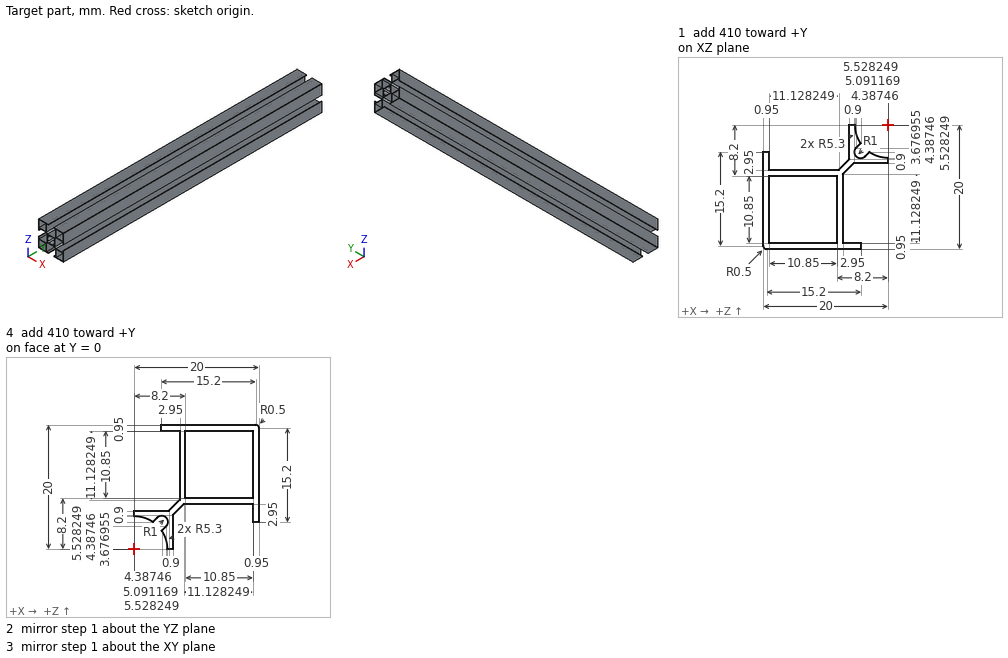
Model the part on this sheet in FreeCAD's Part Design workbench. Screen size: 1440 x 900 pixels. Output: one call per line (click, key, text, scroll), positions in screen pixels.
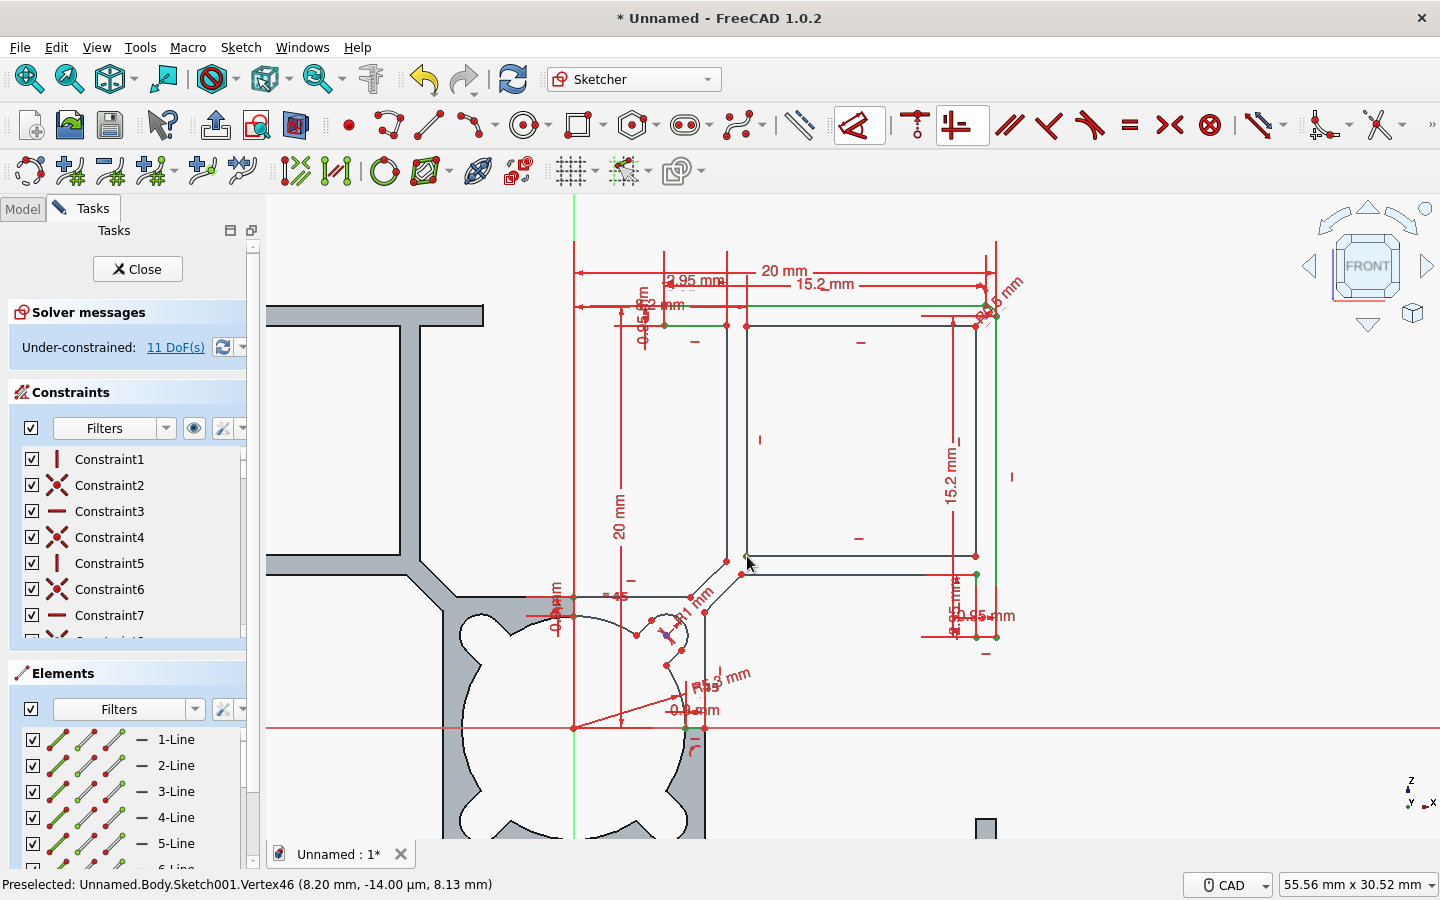
click(880, 126)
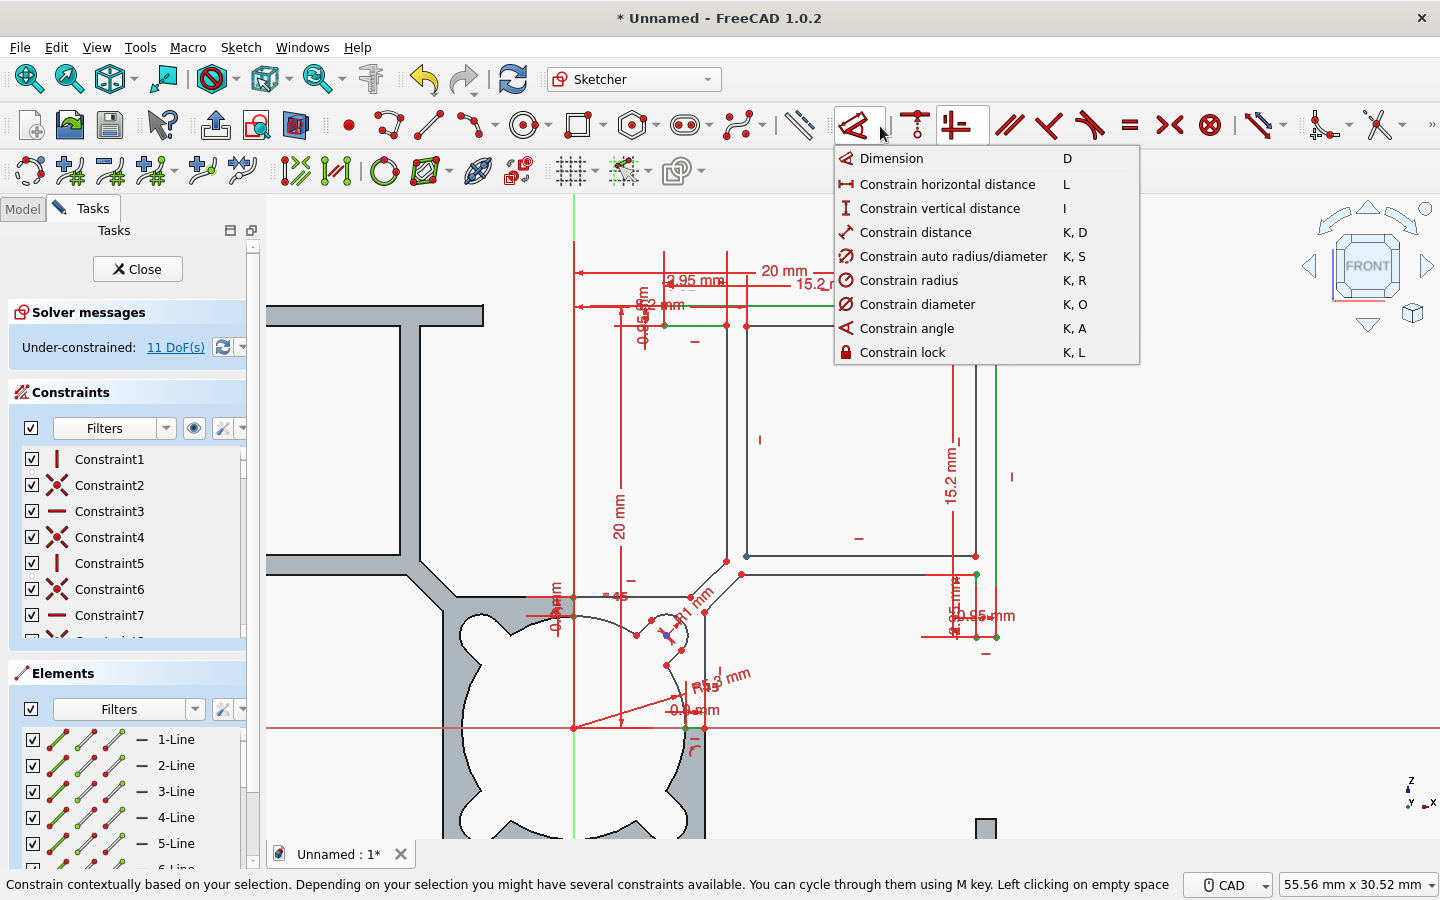
click(987, 208)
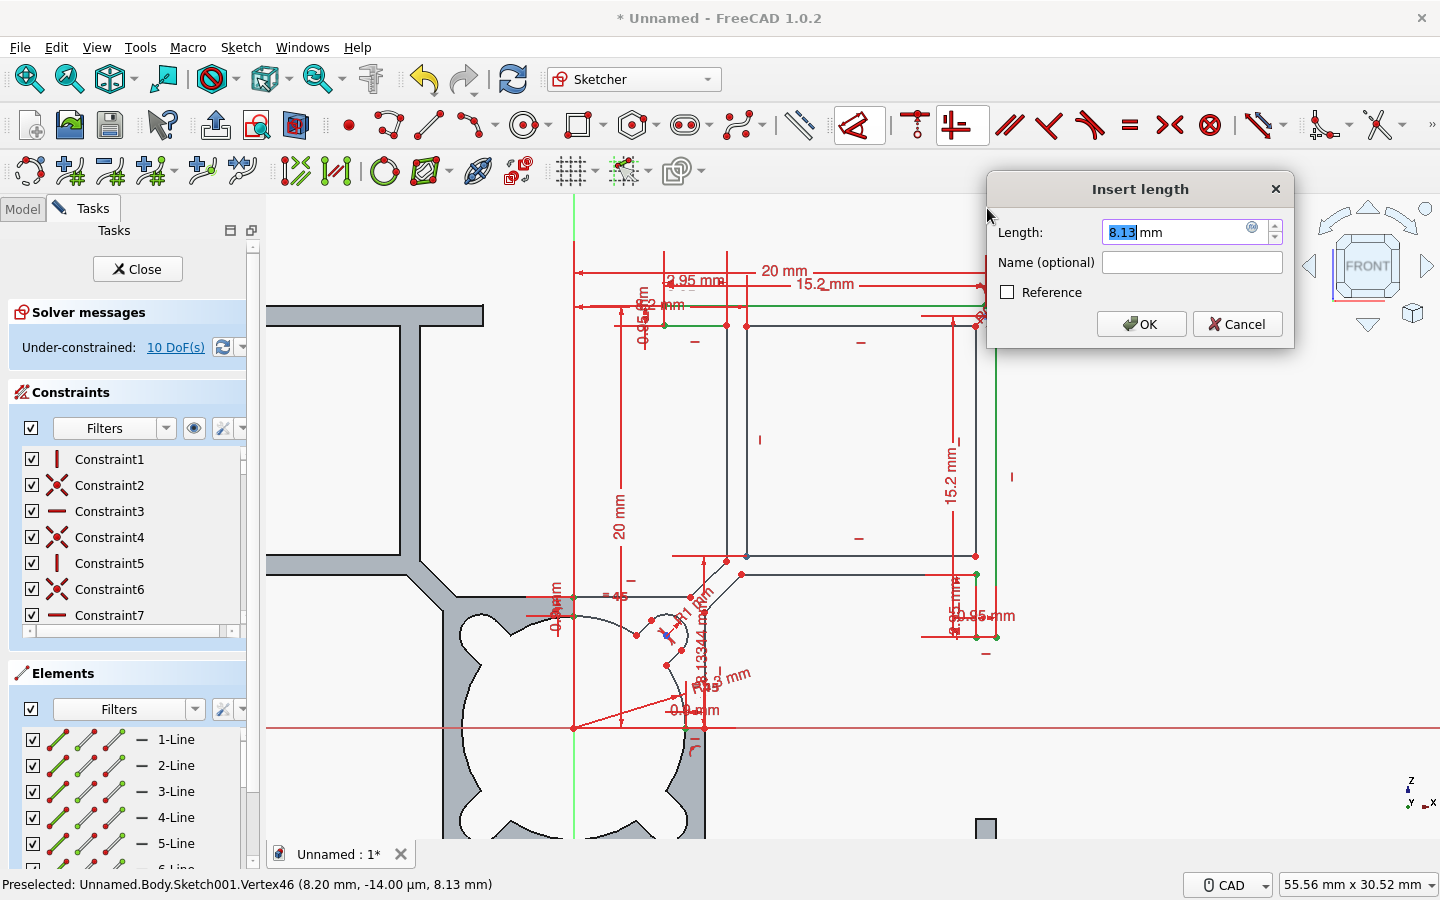
text(8.2)
key(Return)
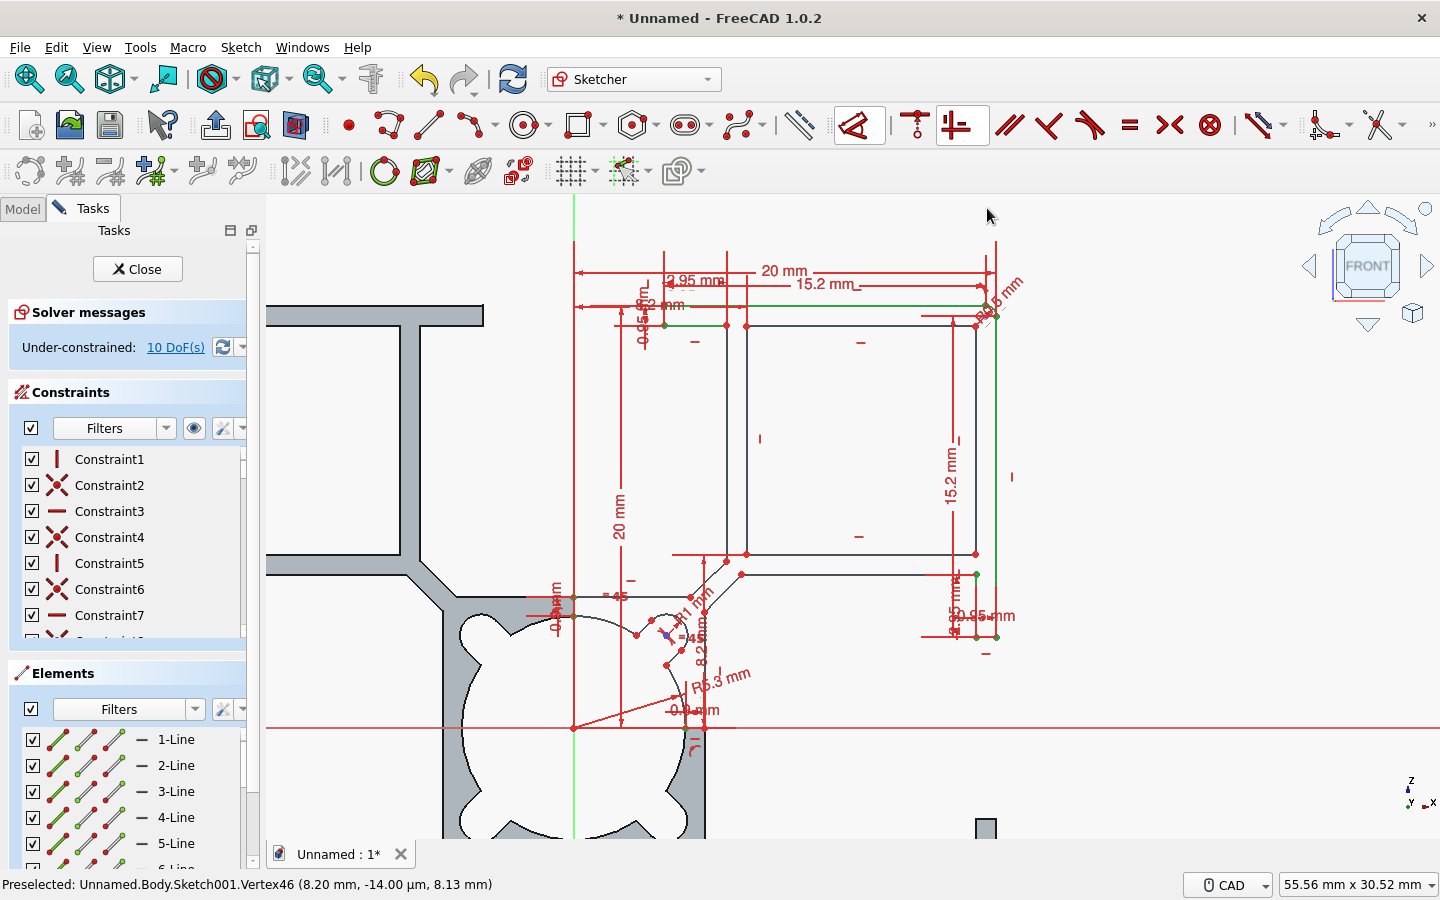
click(747, 395)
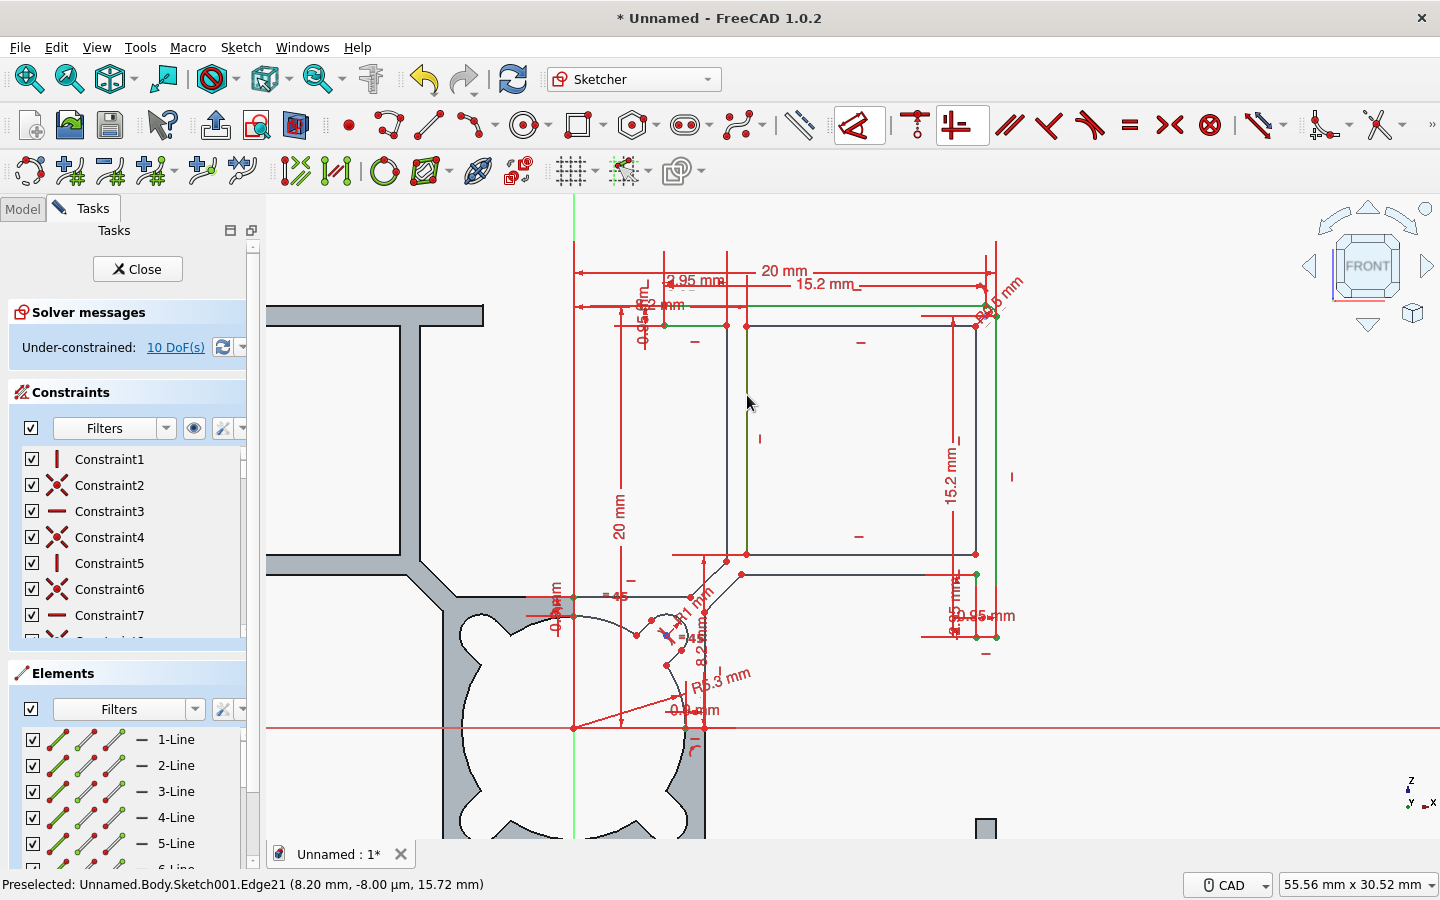
click(880, 126)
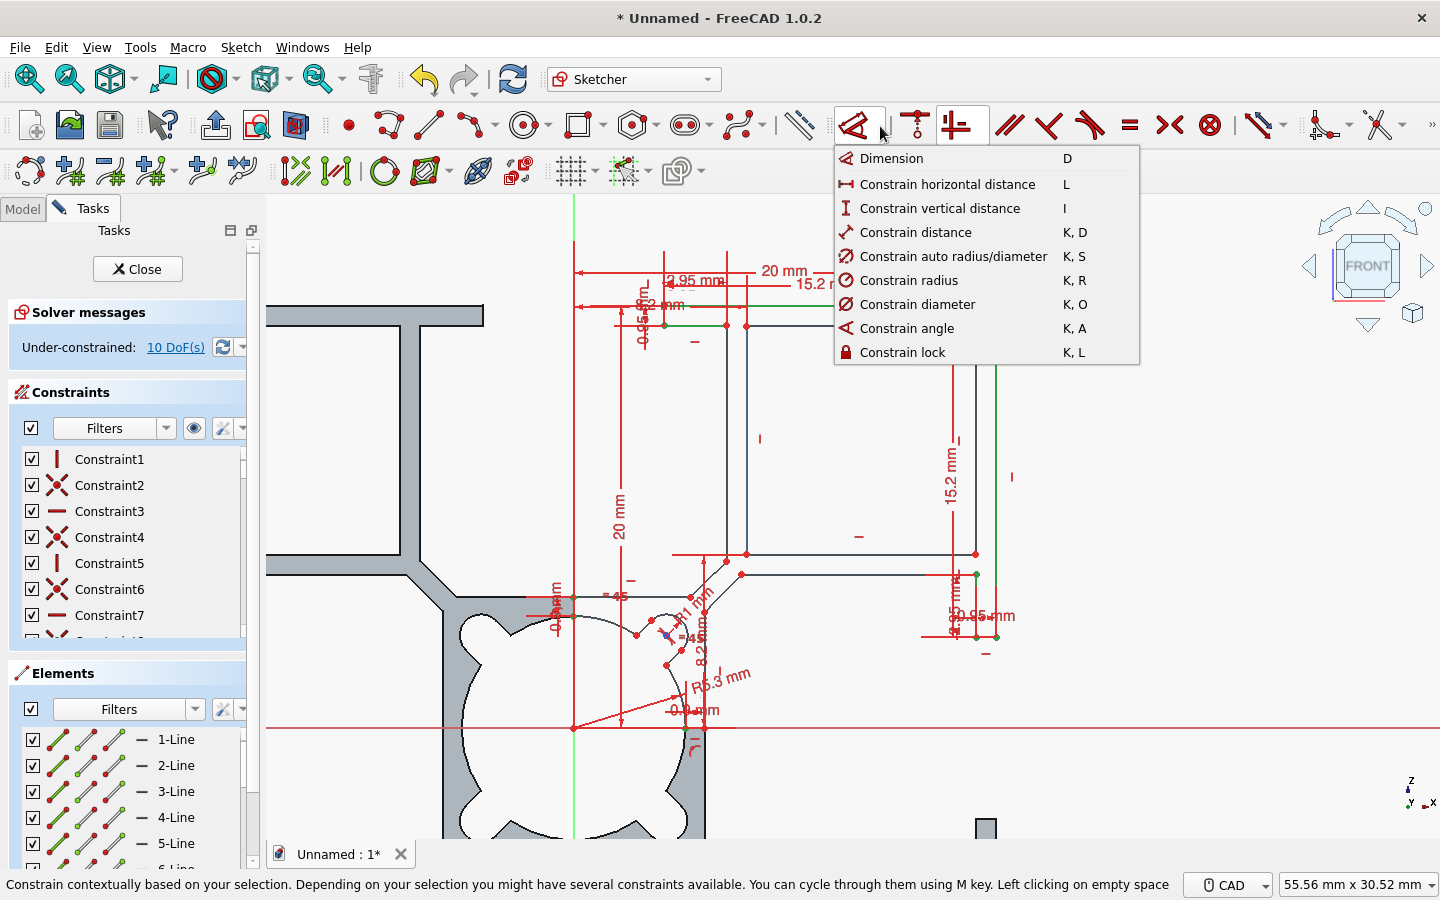
click(987, 208)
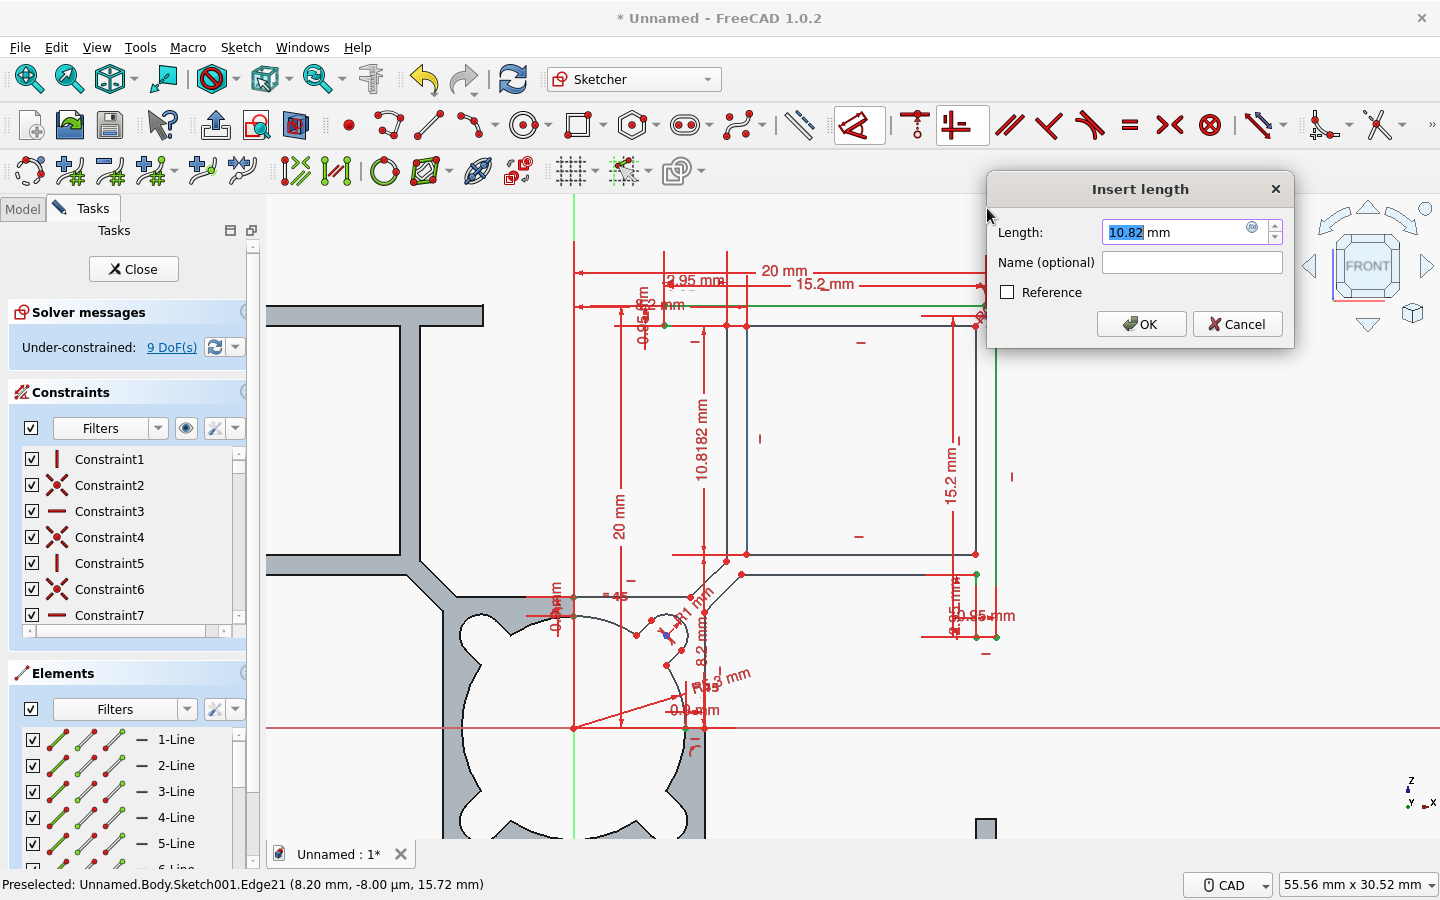
text(10.85)
key(Return)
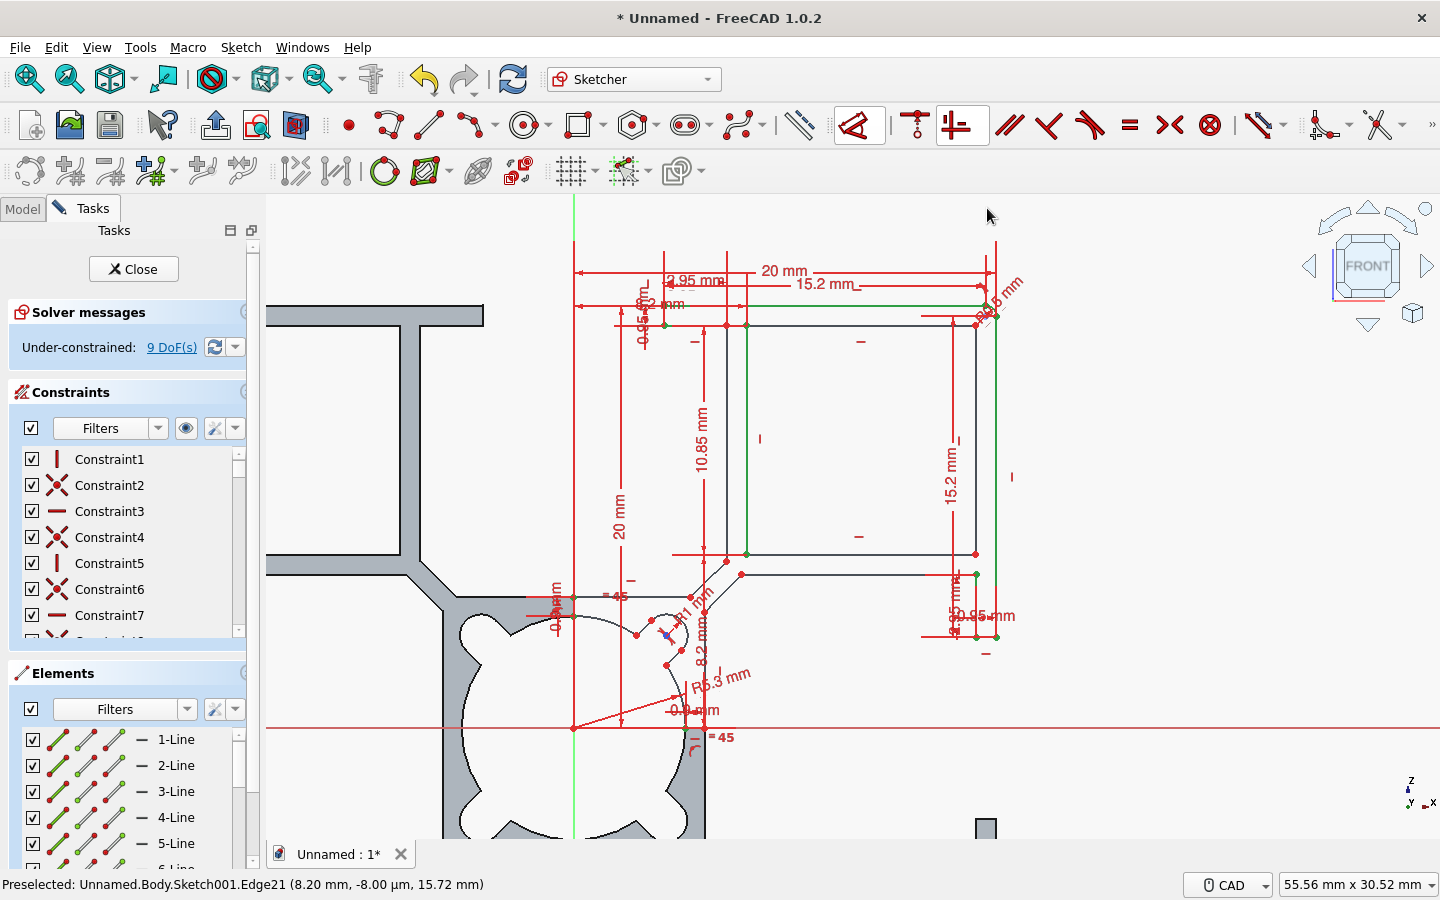
click(816, 555)